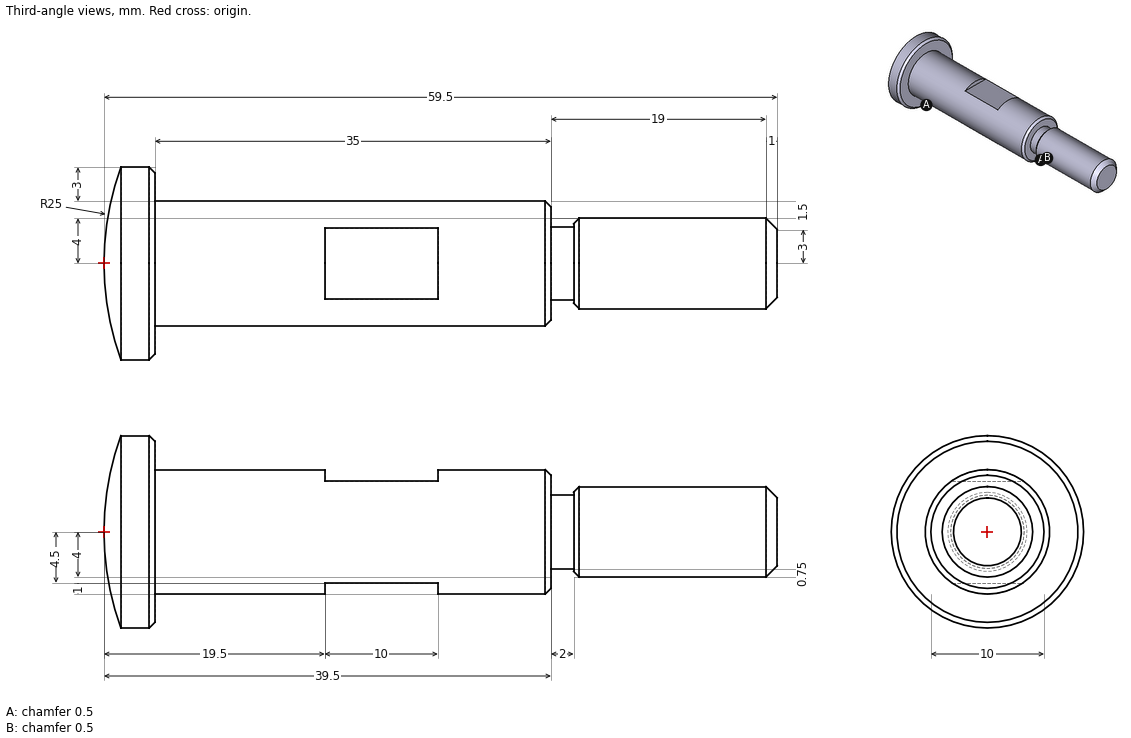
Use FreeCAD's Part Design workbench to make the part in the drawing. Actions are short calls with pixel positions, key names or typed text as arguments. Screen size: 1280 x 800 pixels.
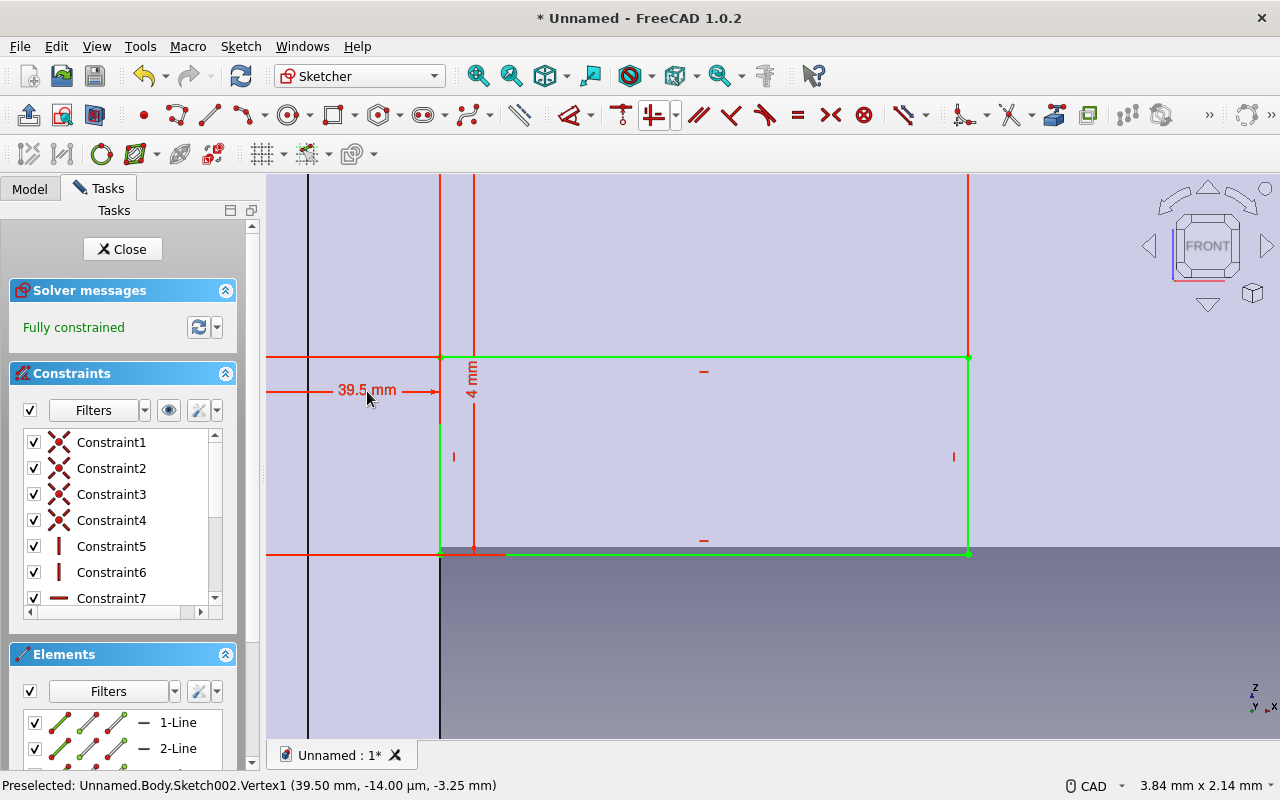
click(123, 249)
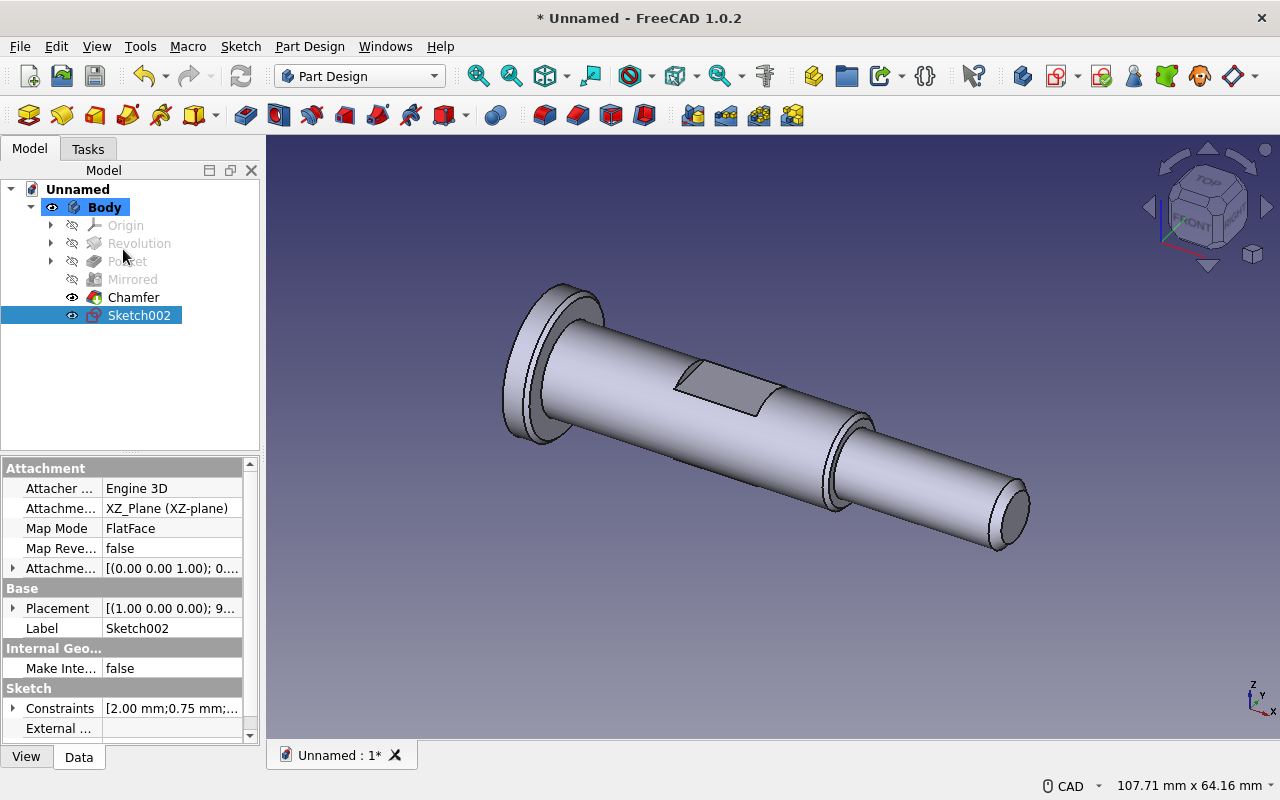
click(312, 116)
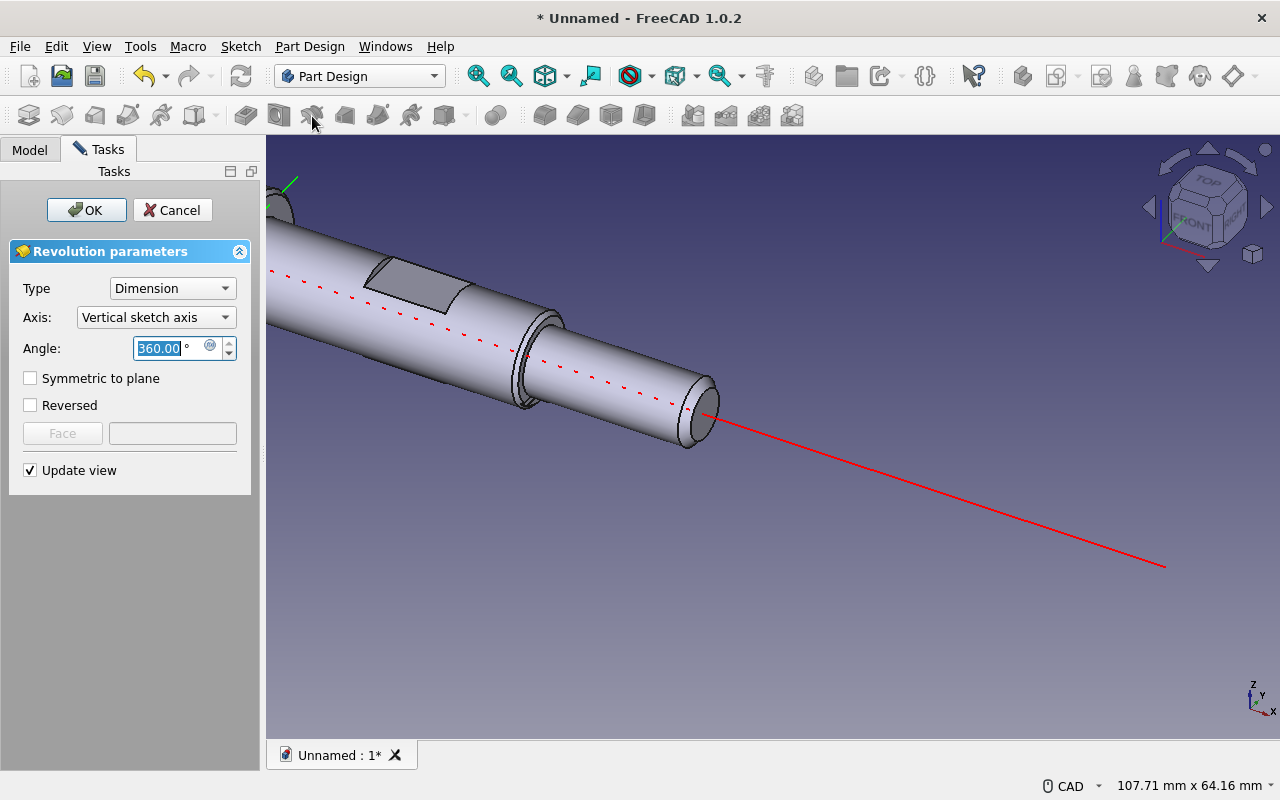
click(157, 318)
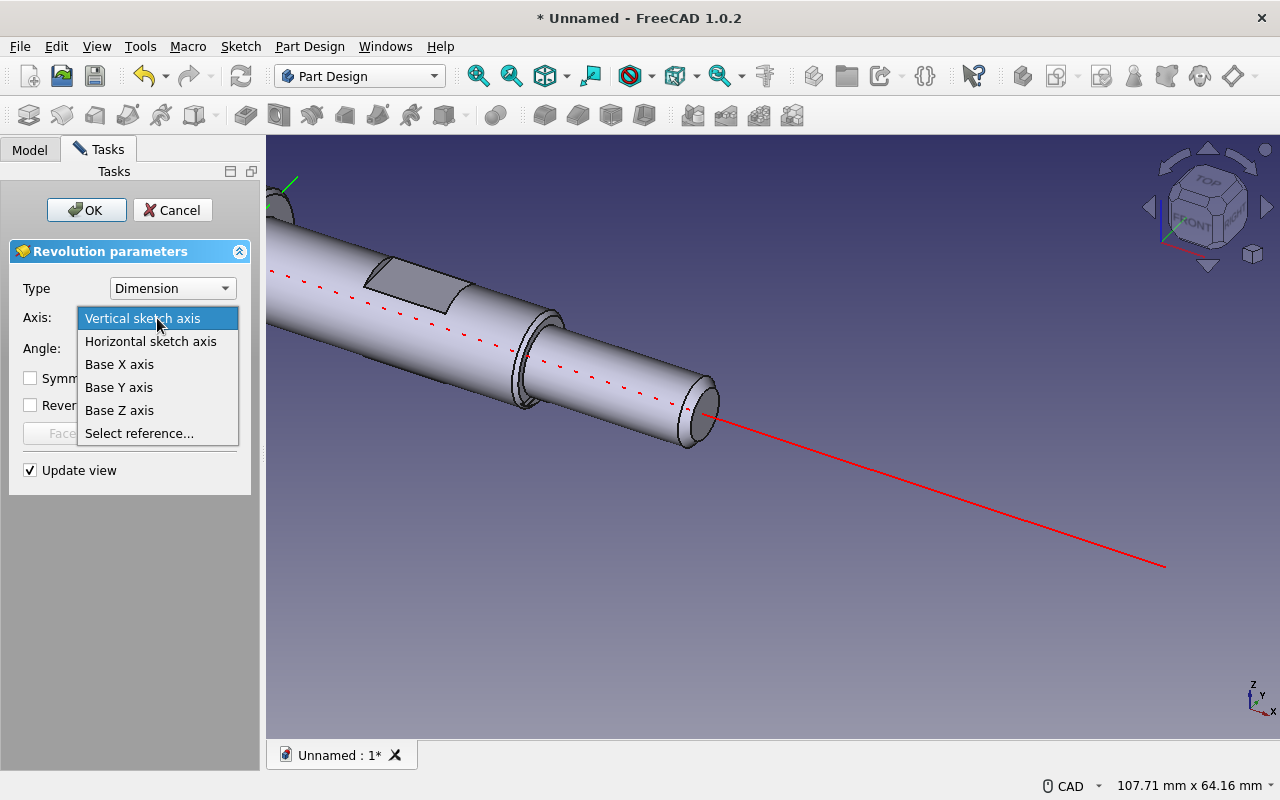
click(156, 342)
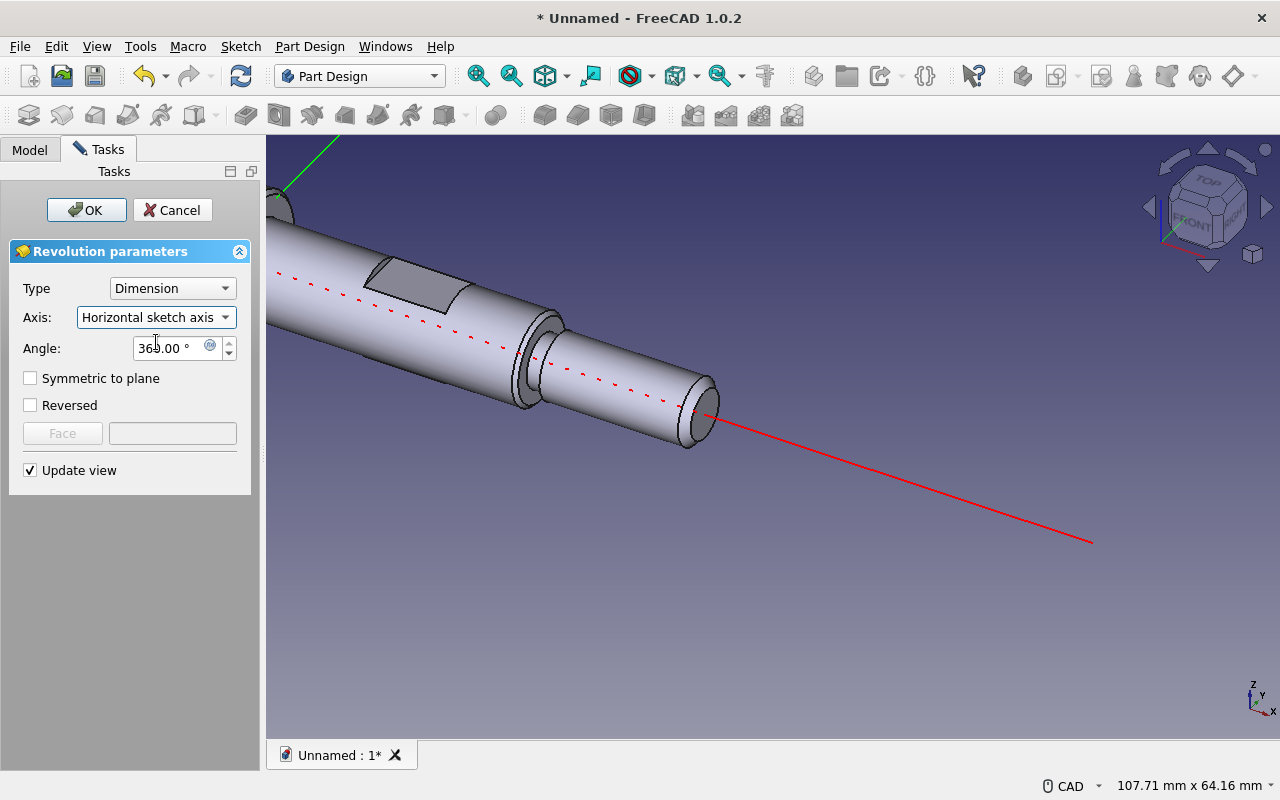
click(87, 210)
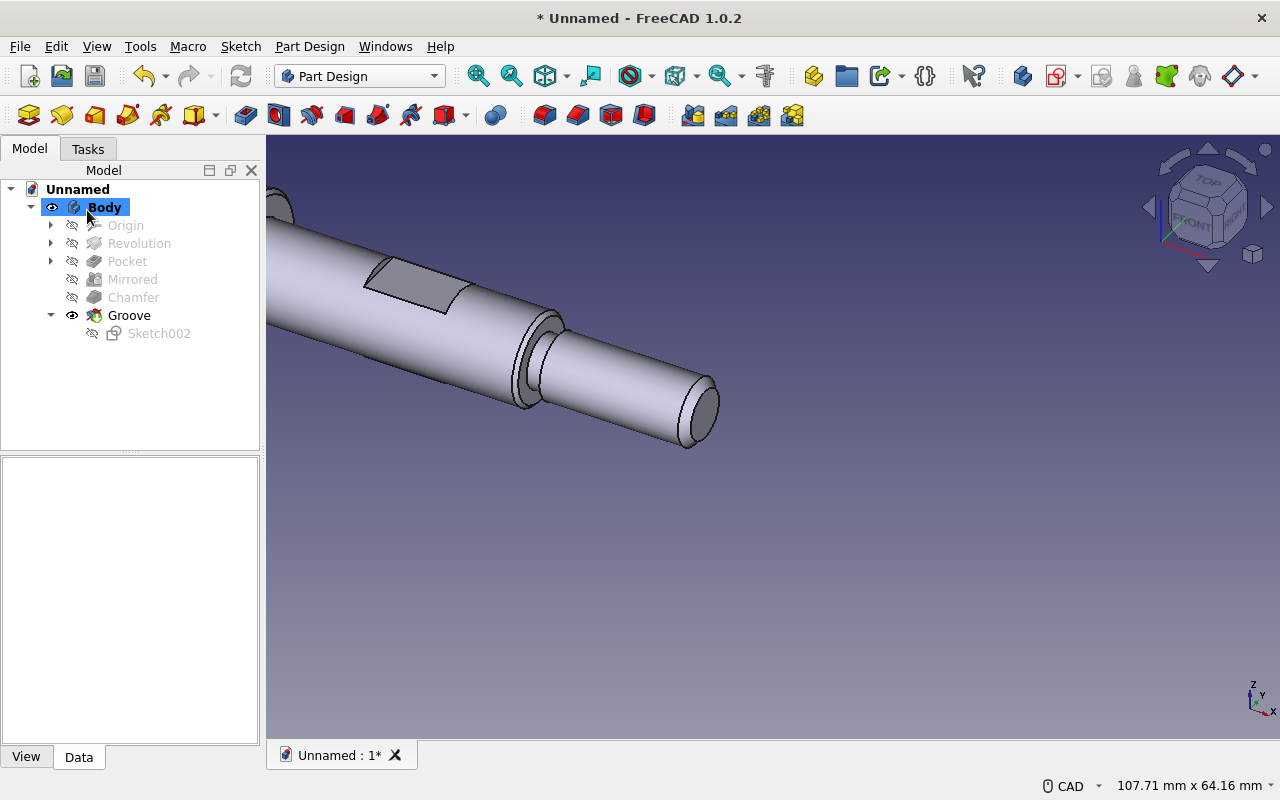
click(479, 76)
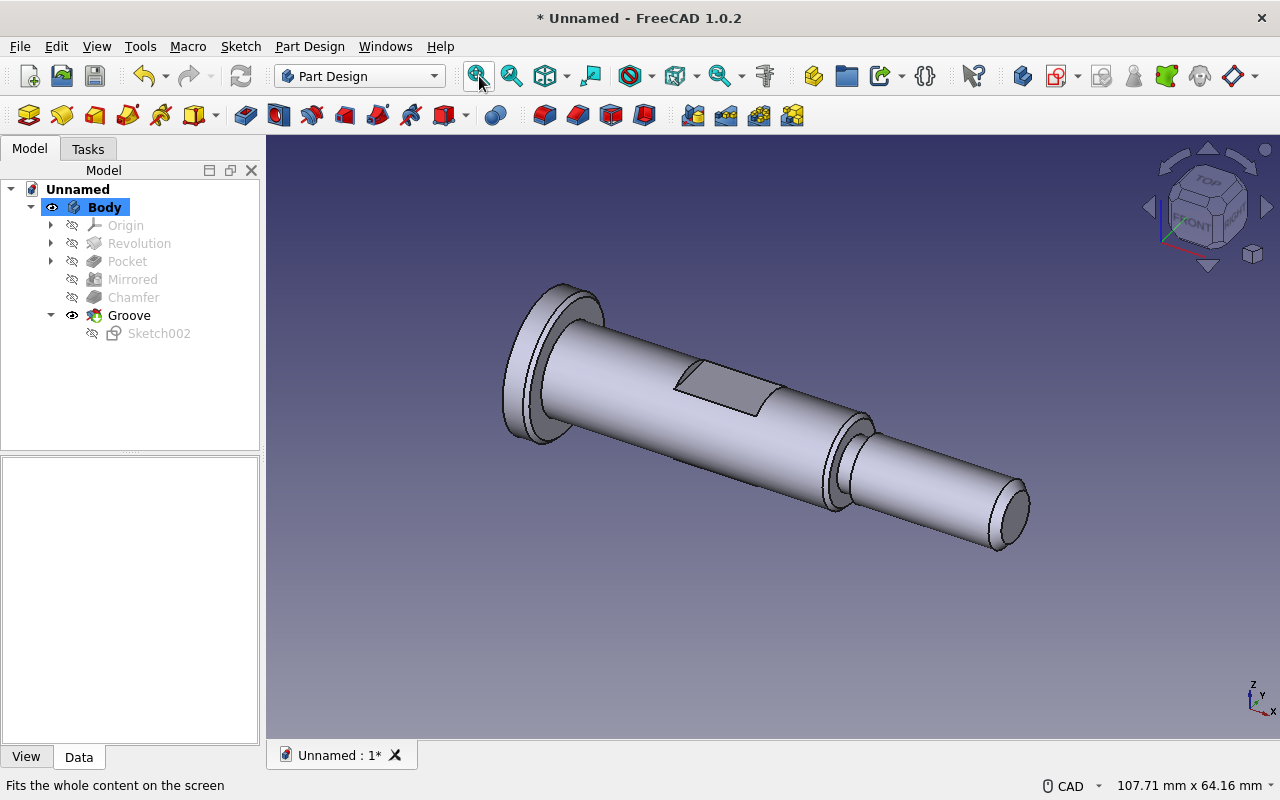
key(0)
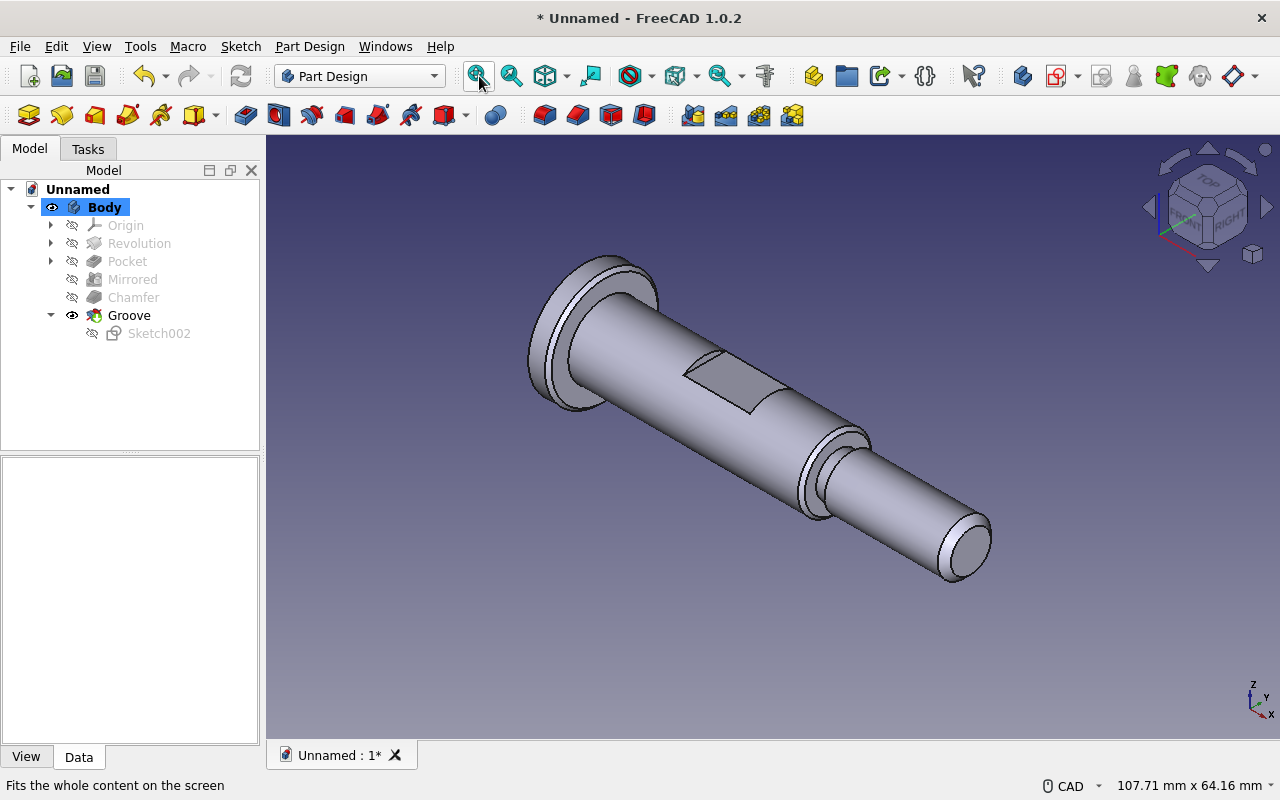
key(2)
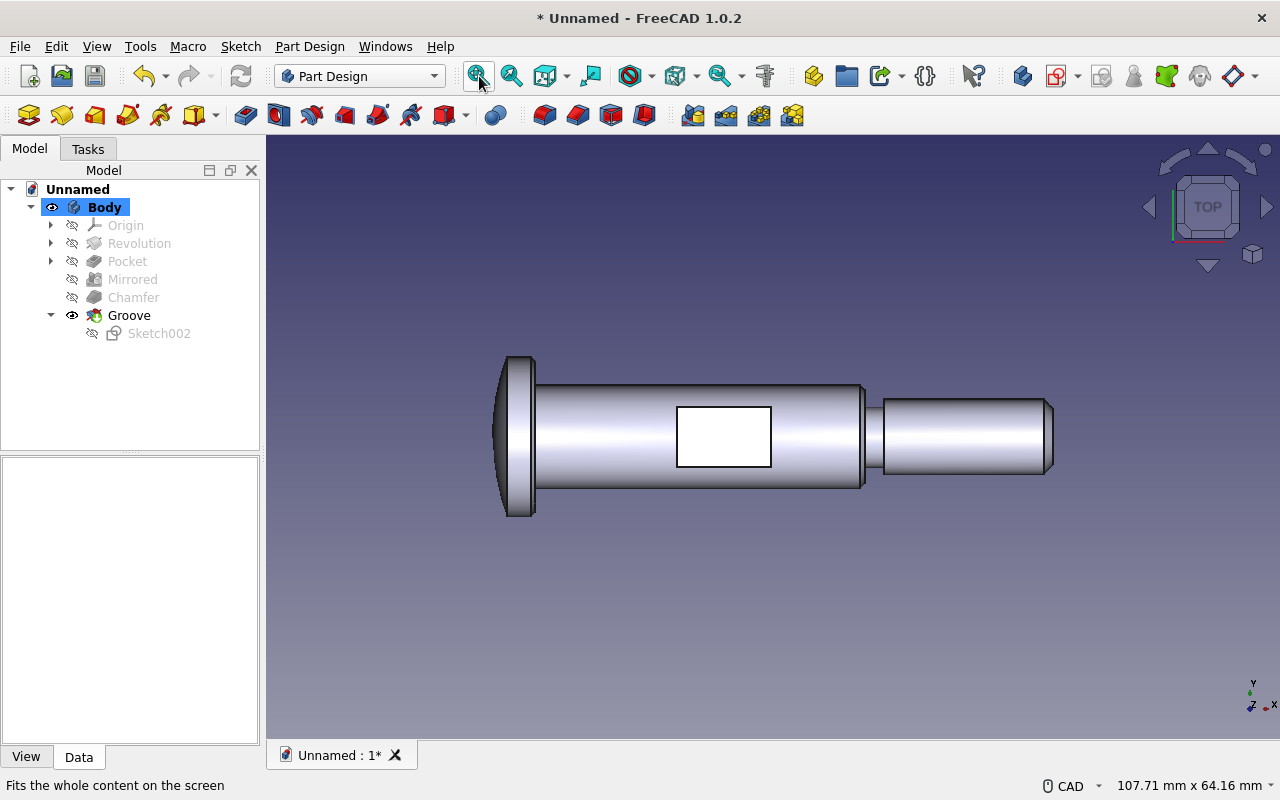
key(1)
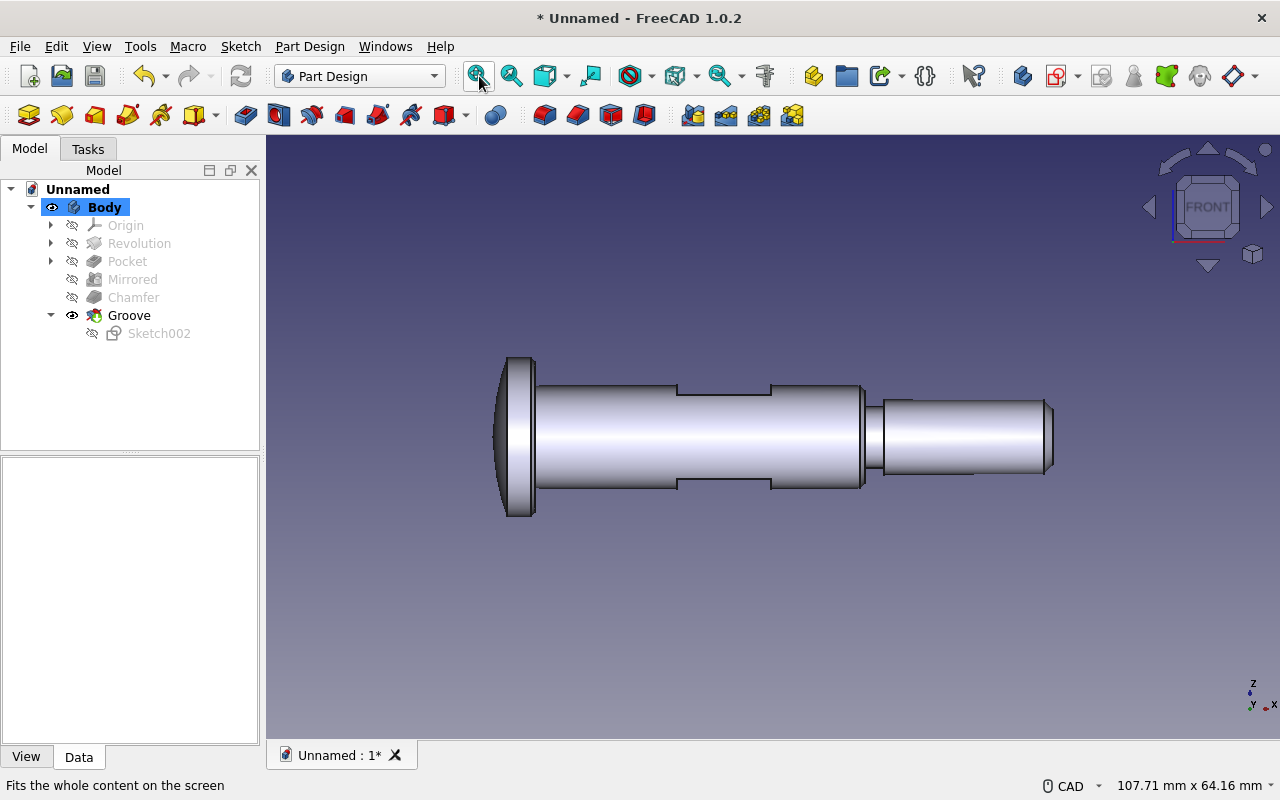
key(3)